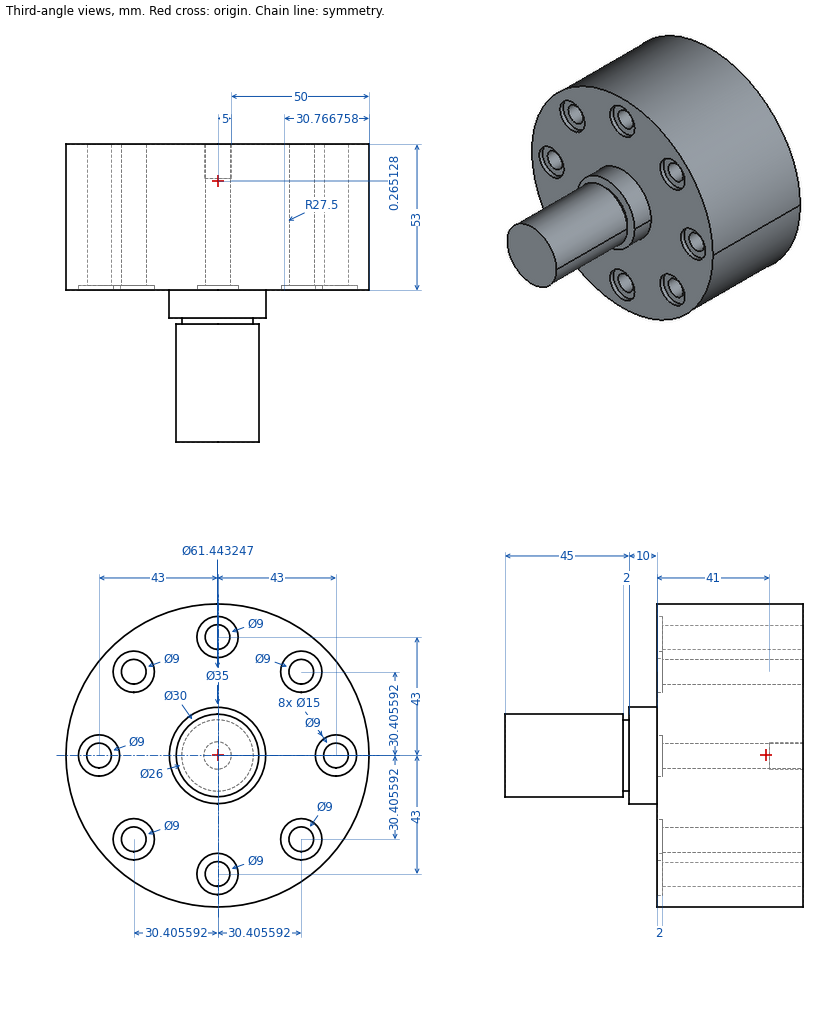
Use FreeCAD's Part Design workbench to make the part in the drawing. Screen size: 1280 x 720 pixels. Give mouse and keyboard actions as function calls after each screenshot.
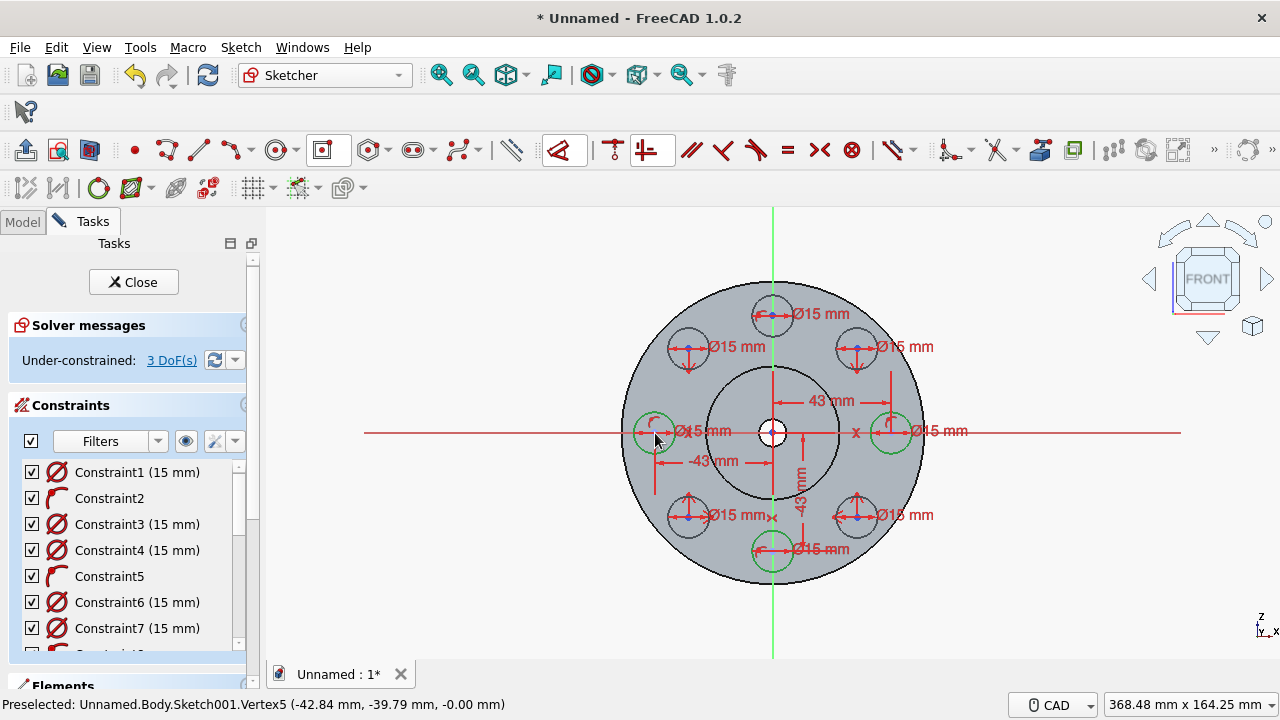
click(773, 316)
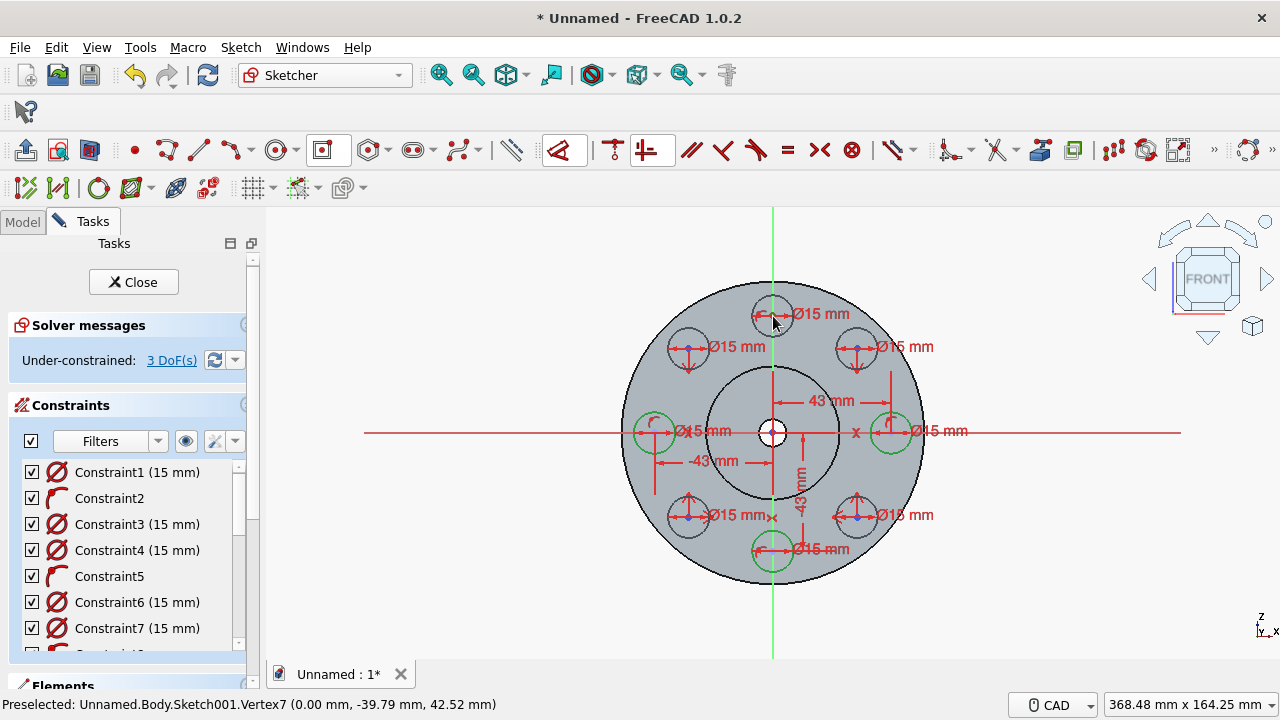
click(582, 150)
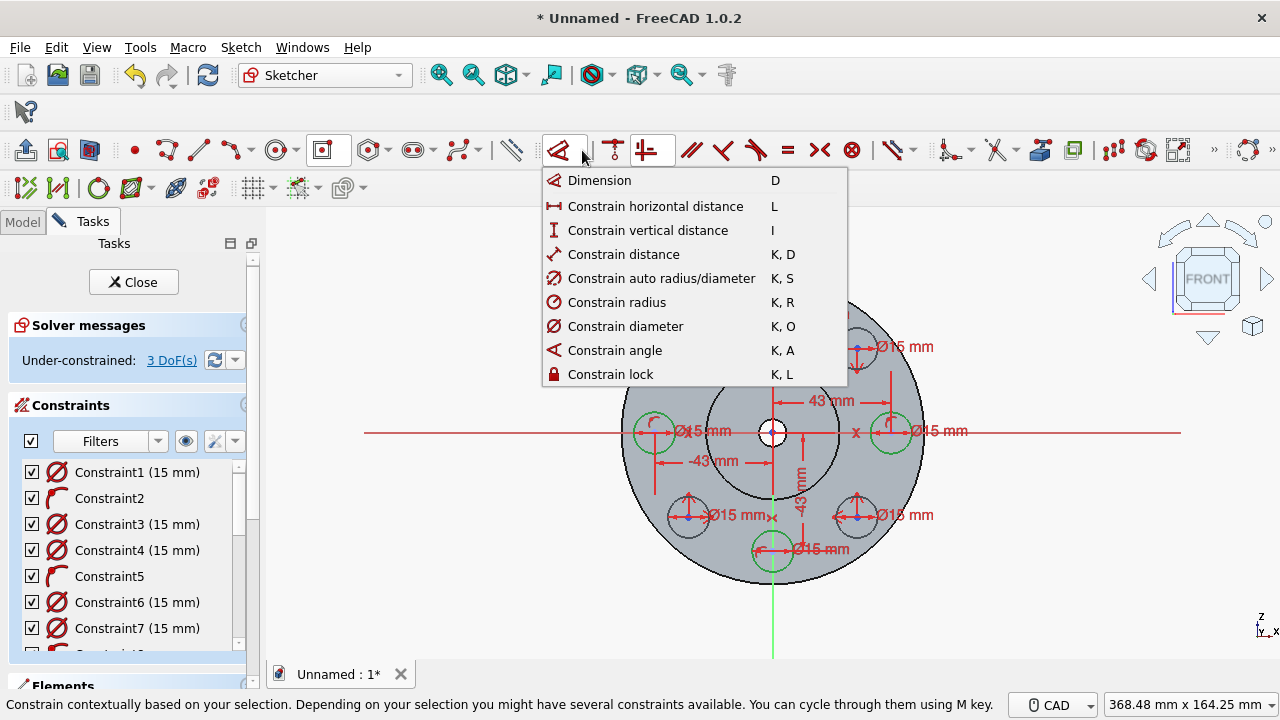
click(695, 230)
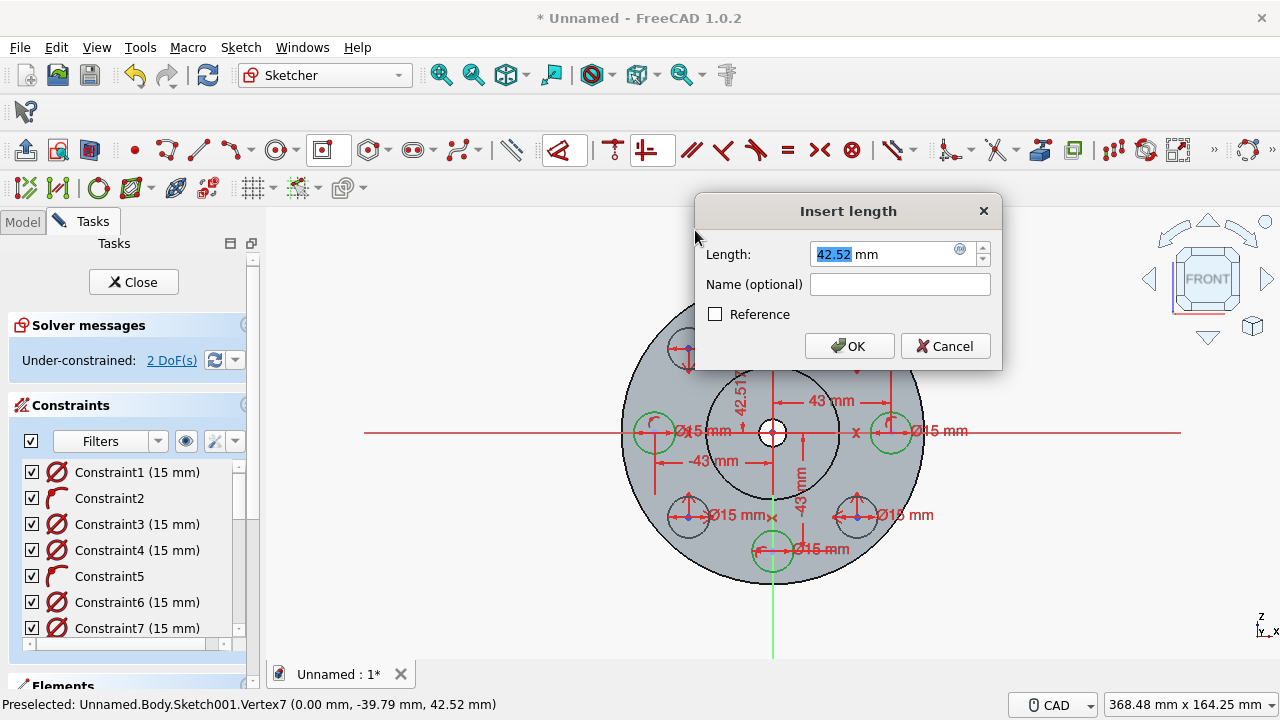
text(43)
key(Return)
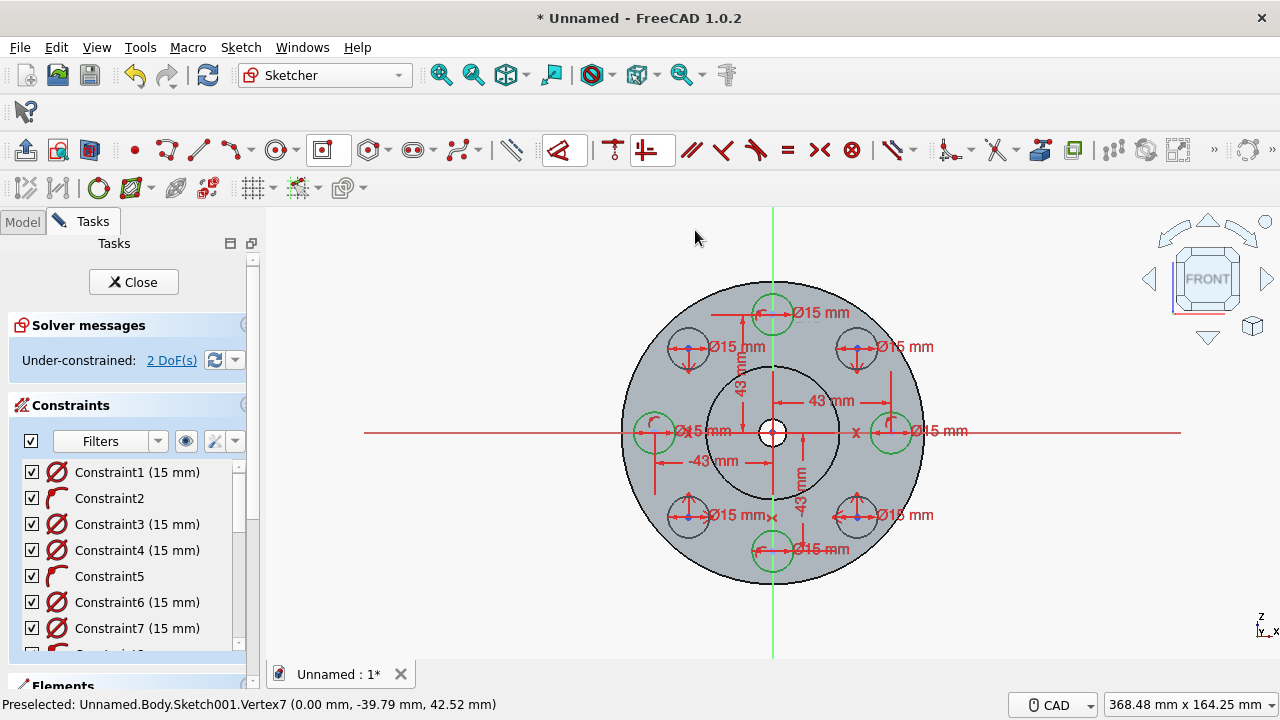
click(857, 517)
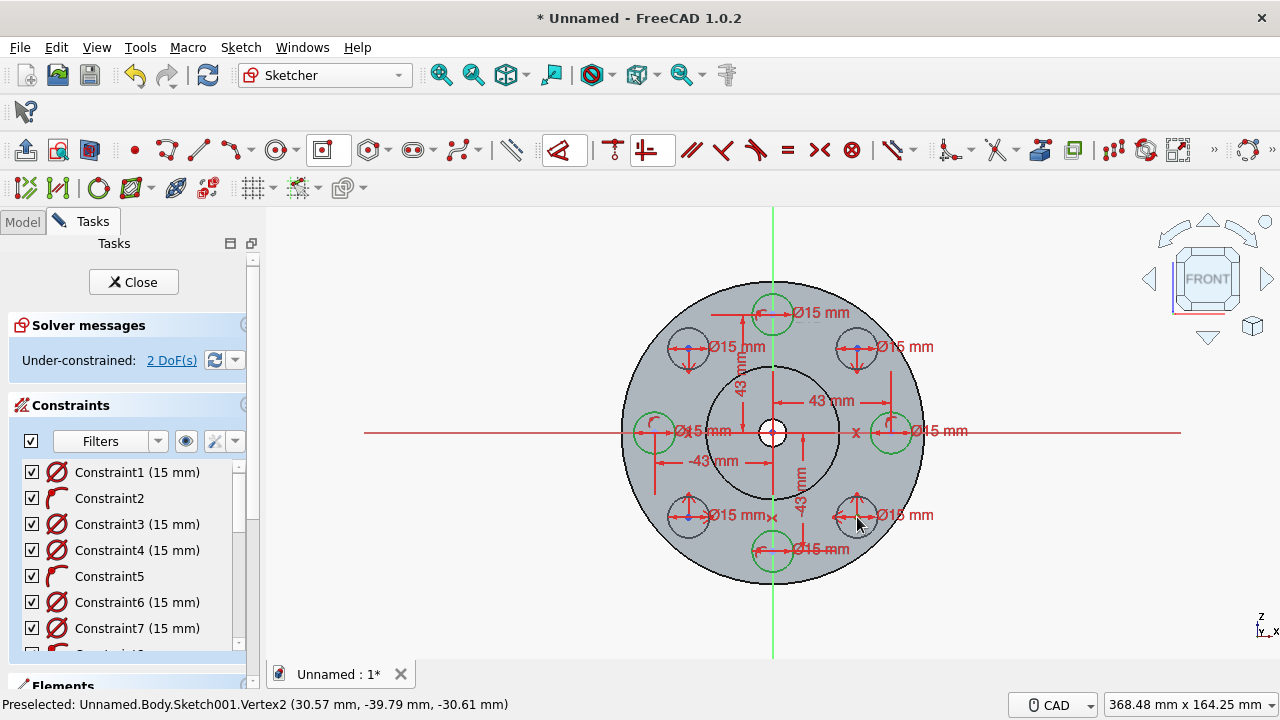
click(582, 150)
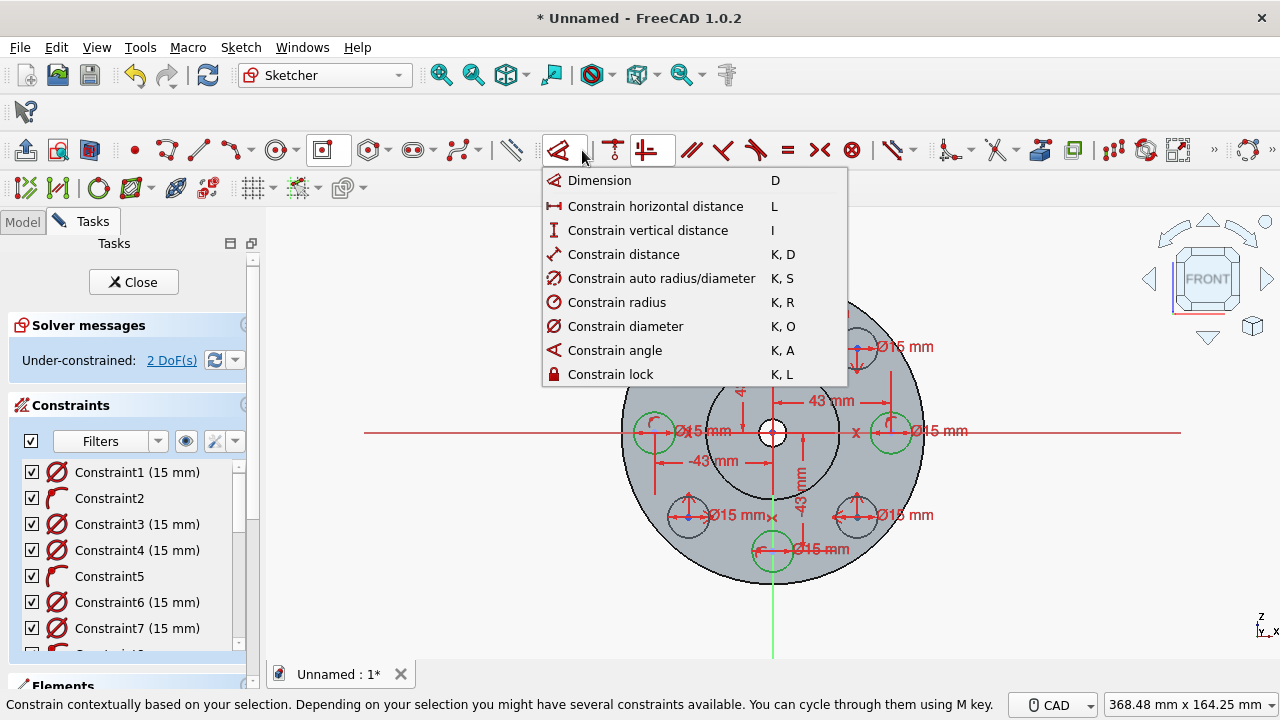
click(695, 206)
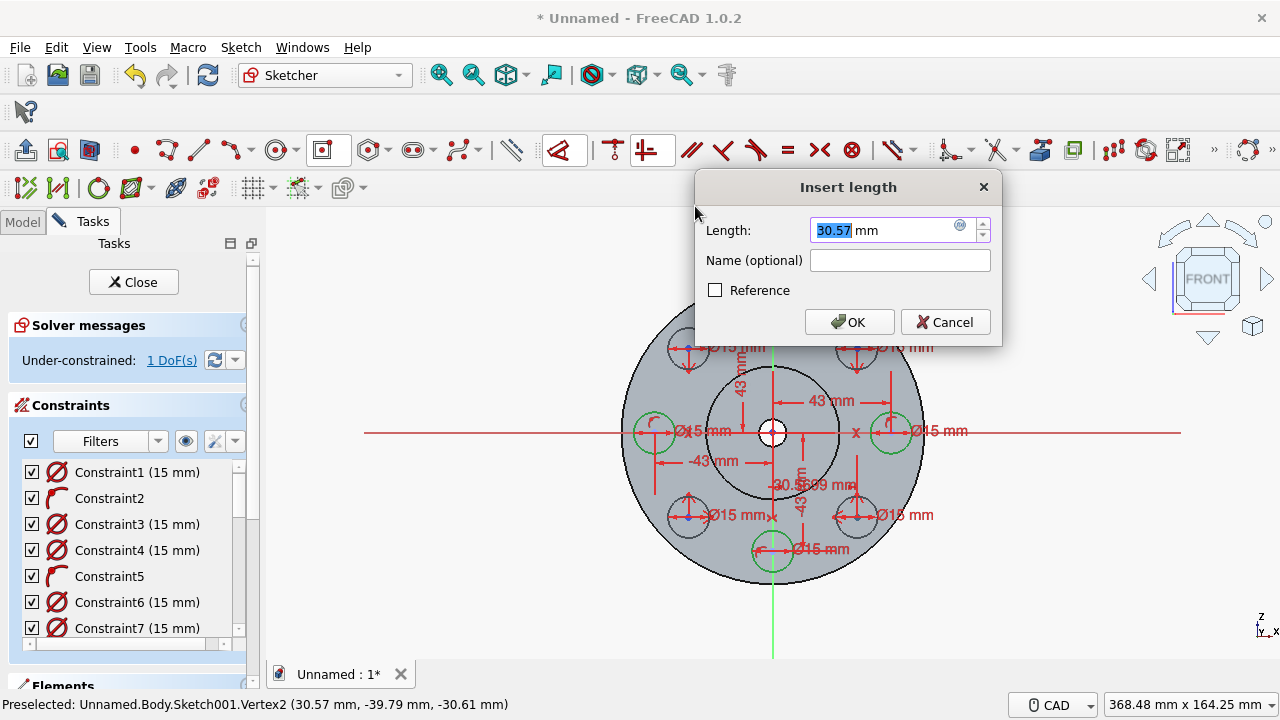
text(30.405592)
key(Return)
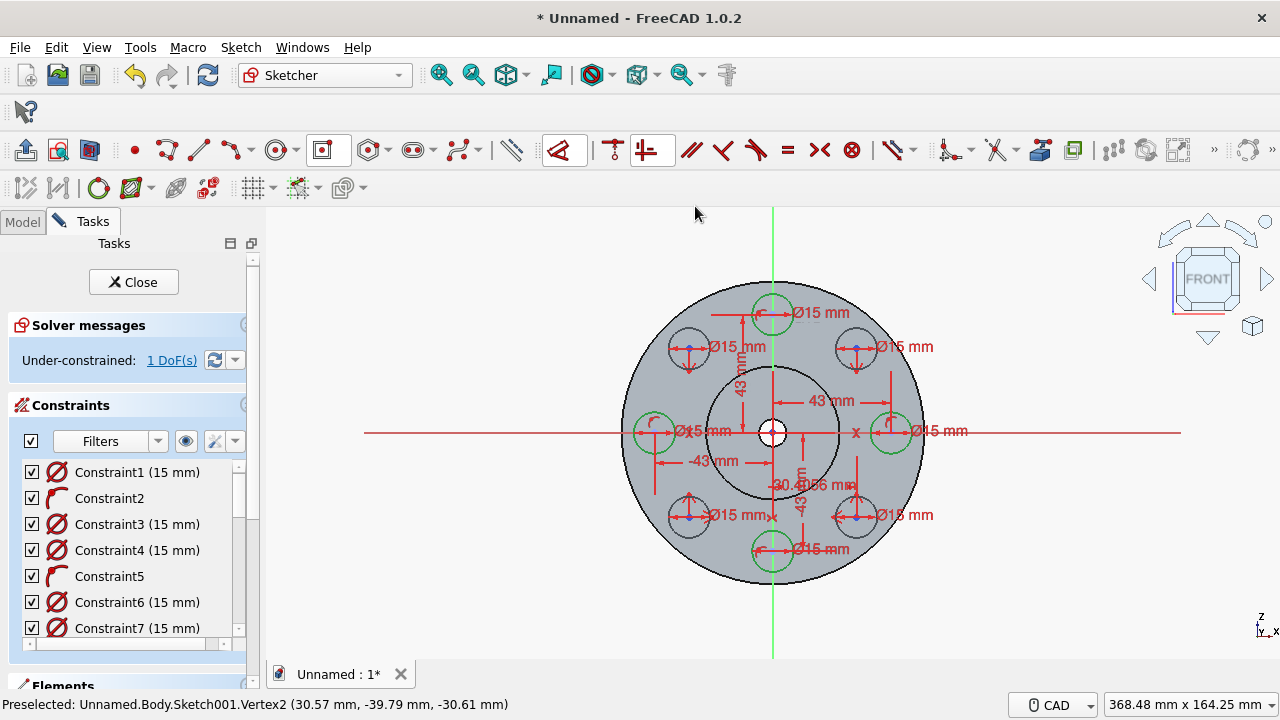
click(857, 517)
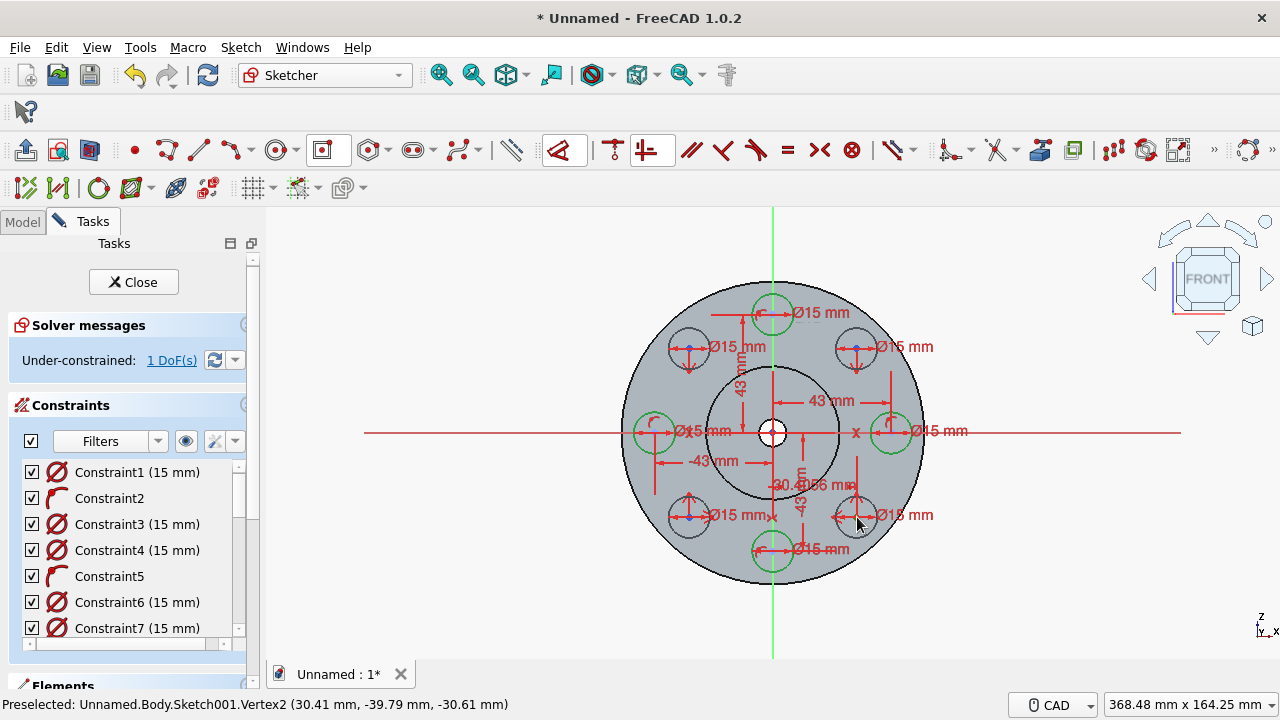
click(582, 150)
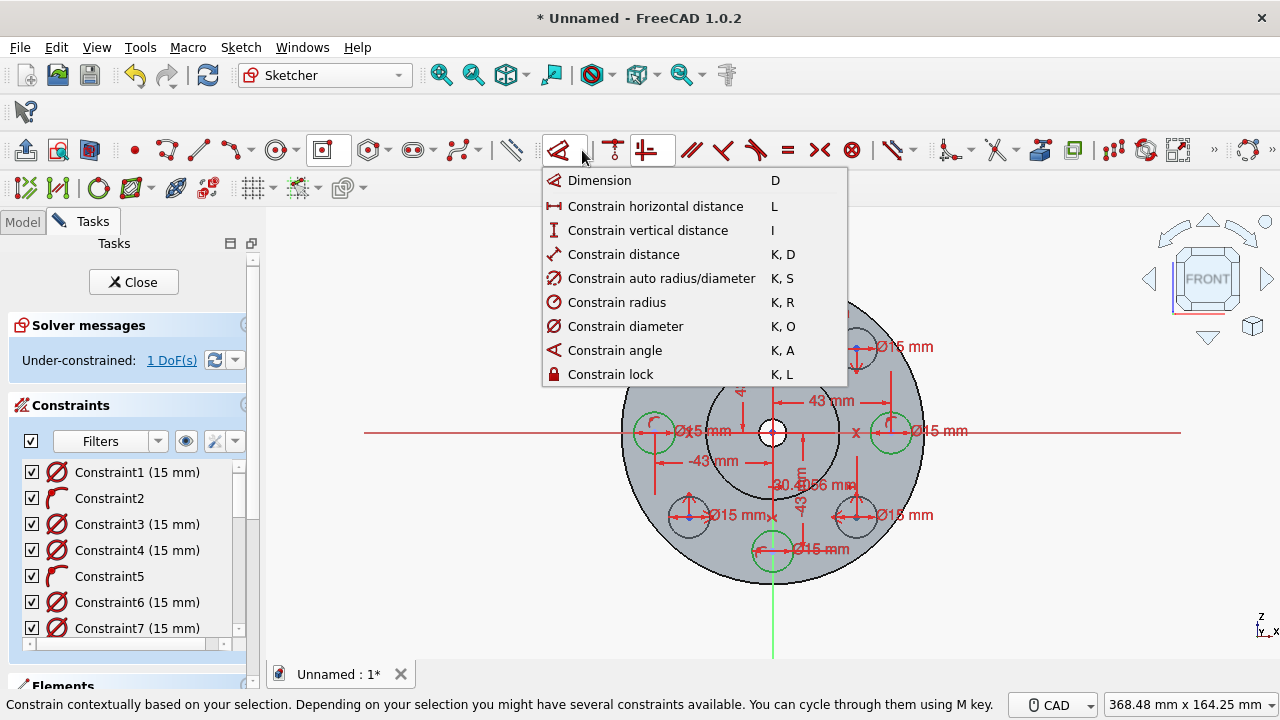
click(695, 230)